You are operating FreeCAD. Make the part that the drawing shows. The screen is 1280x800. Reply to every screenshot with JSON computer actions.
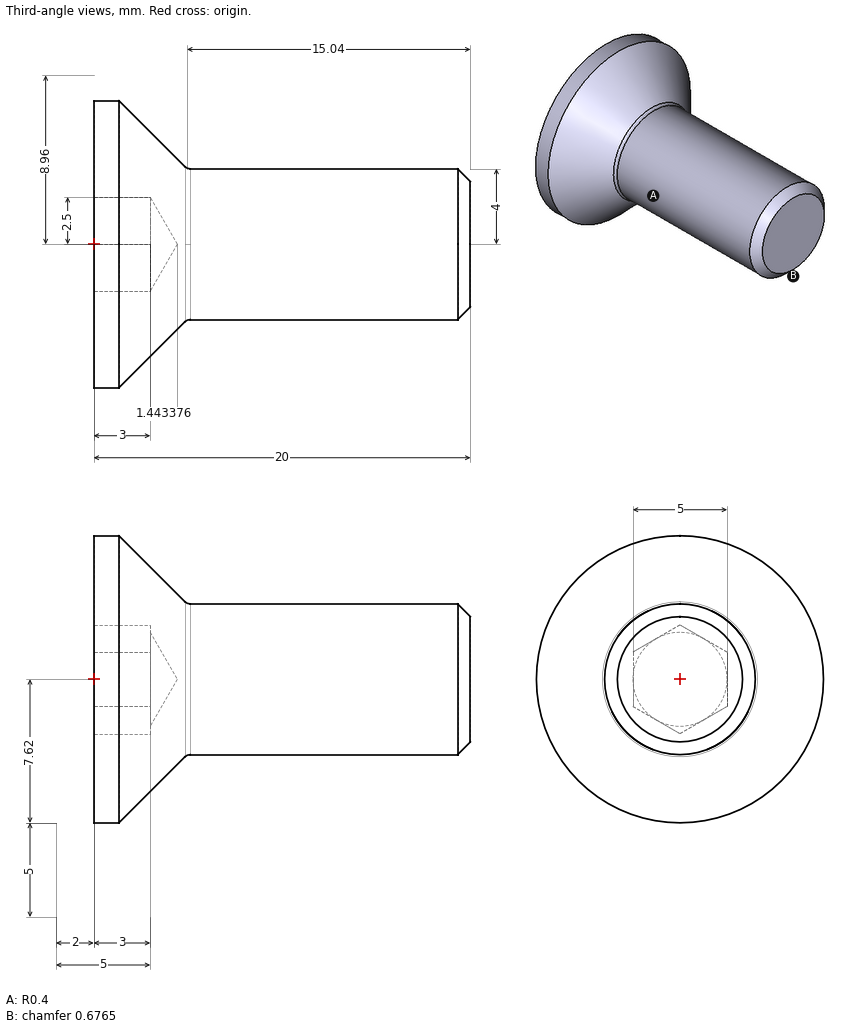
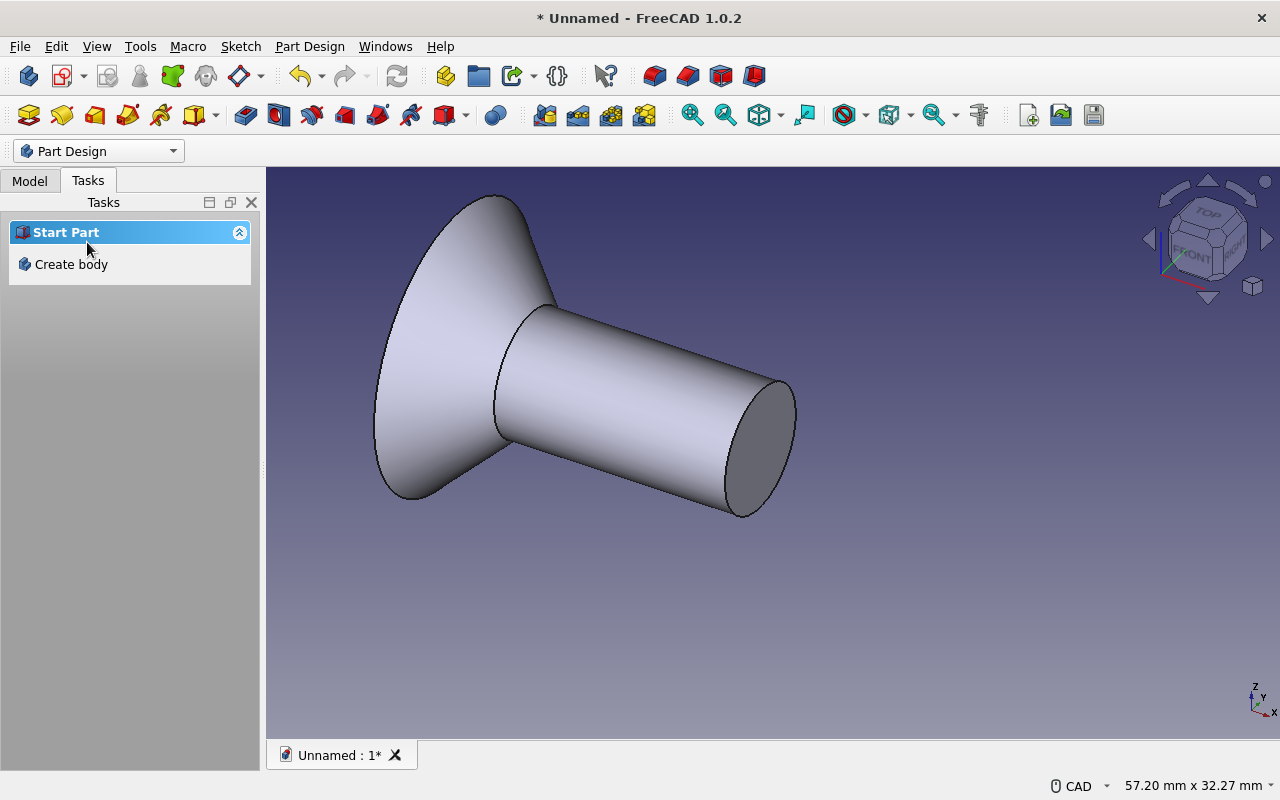
{"action": "left_click", "coordinate": [693, 116]}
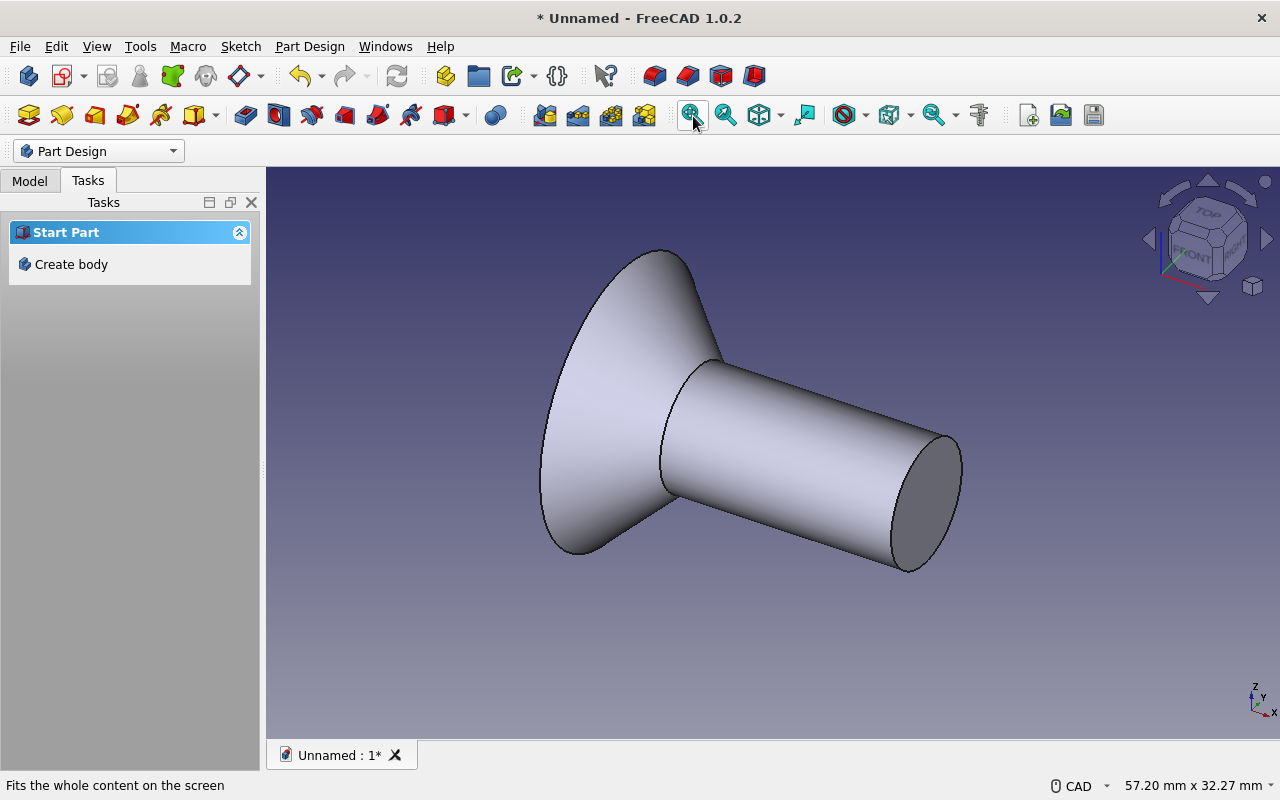
{"action": "key", "text": "0"}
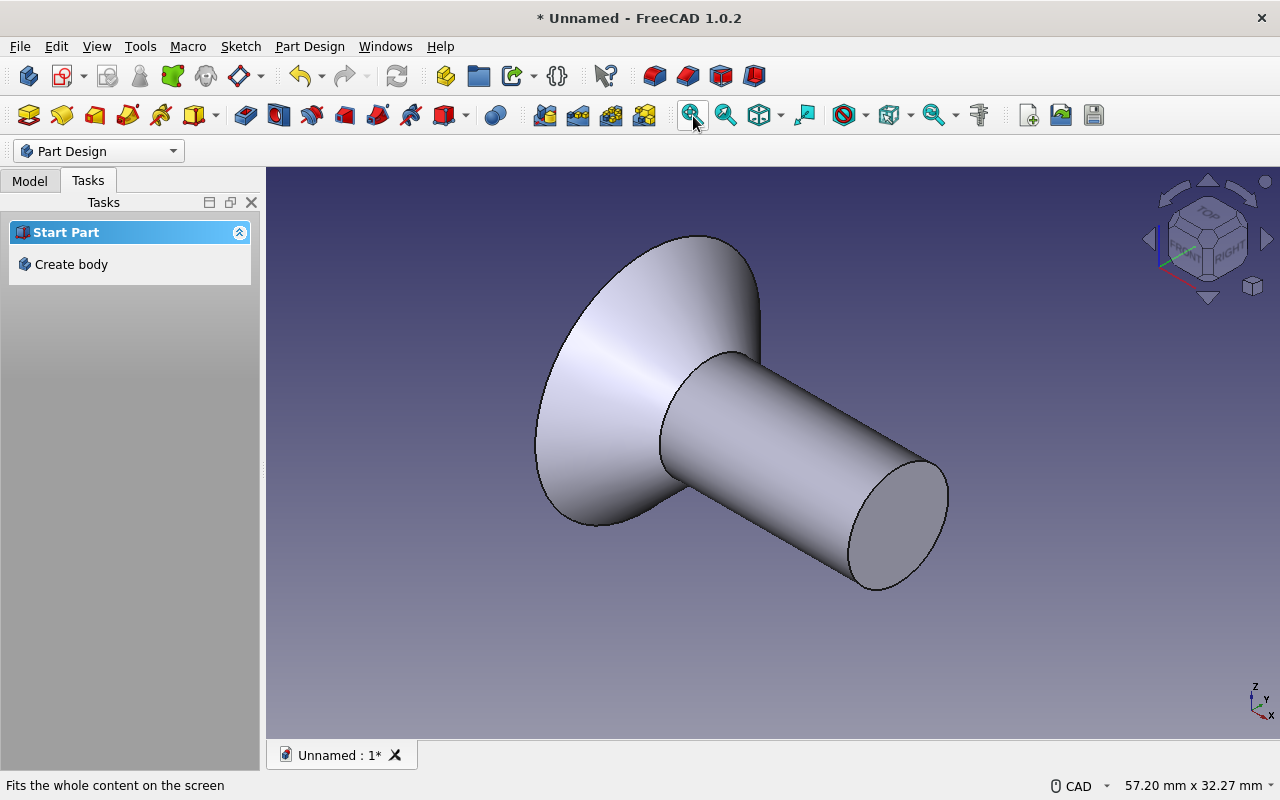
{"action": "key", "text": "2"}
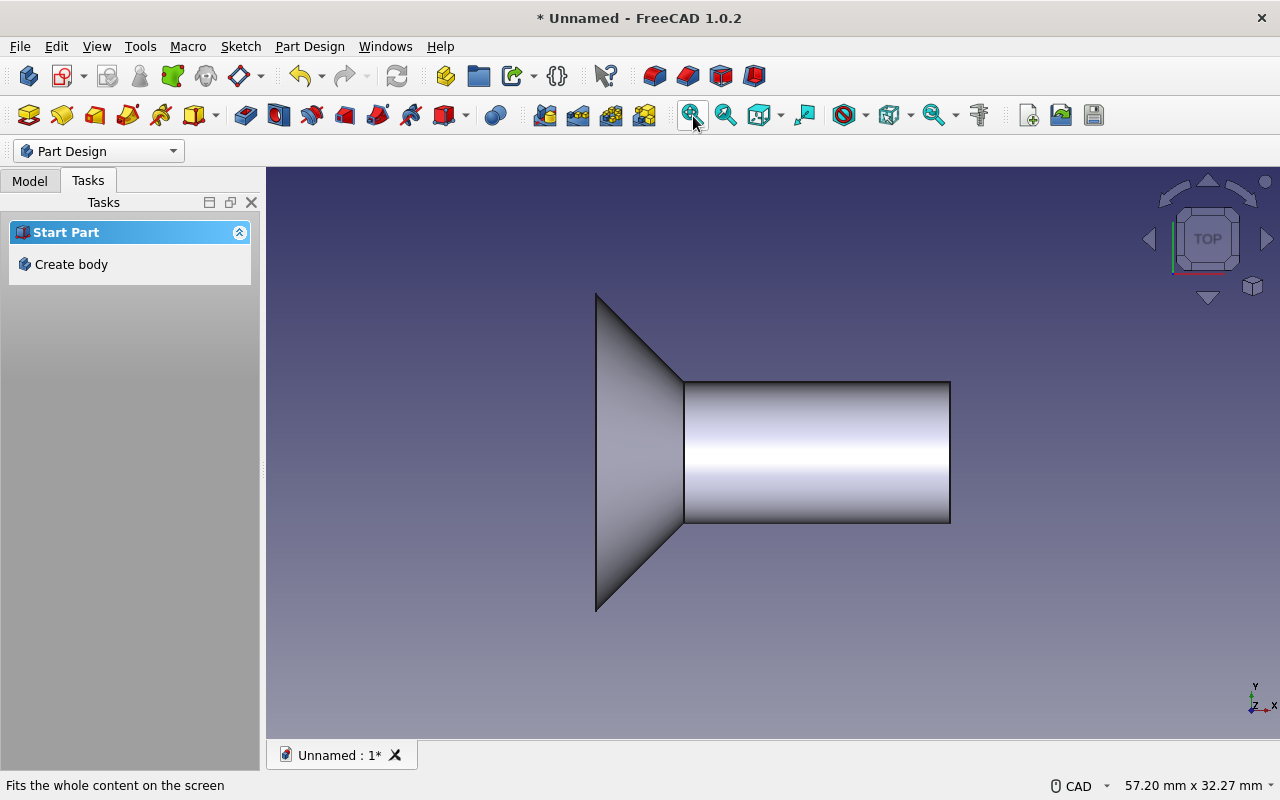
{"action": "left_click", "coordinate": [684, 510]}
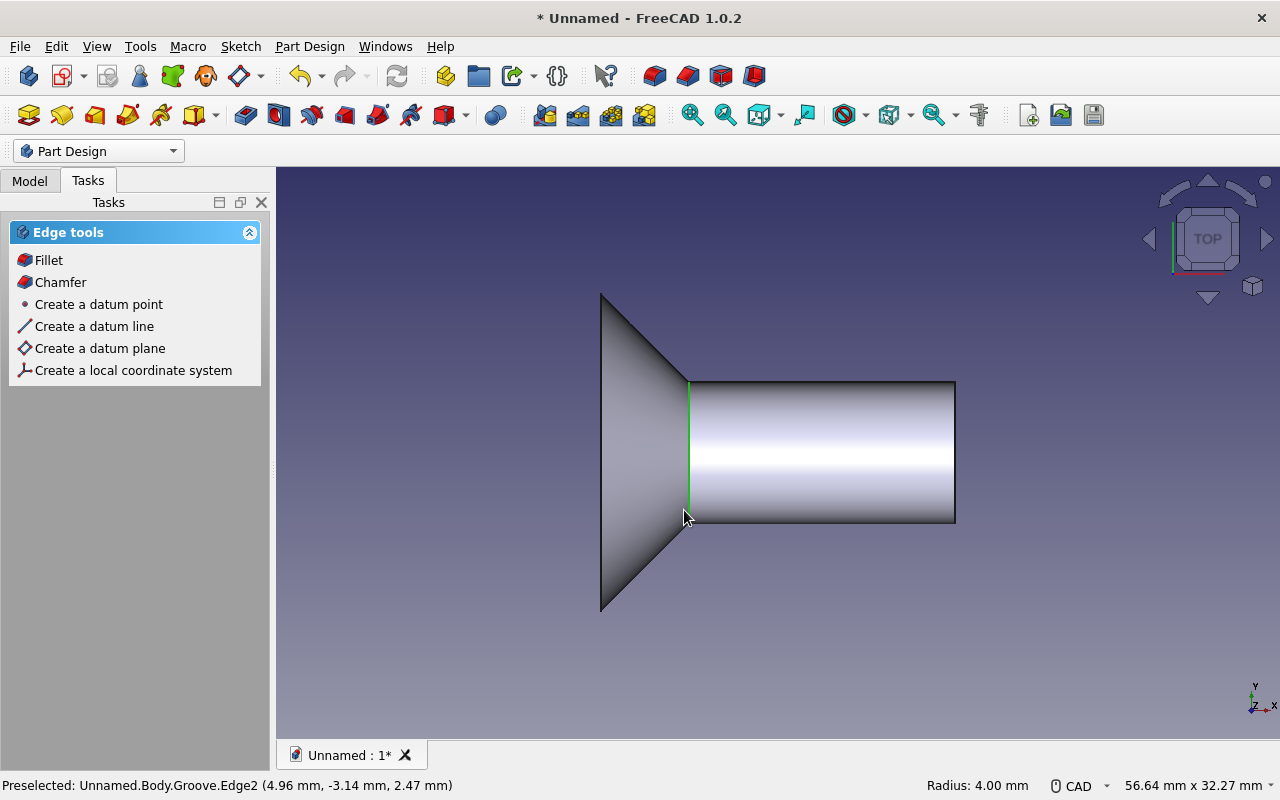
{"action": "left_click", "coordinate": [655, 76]}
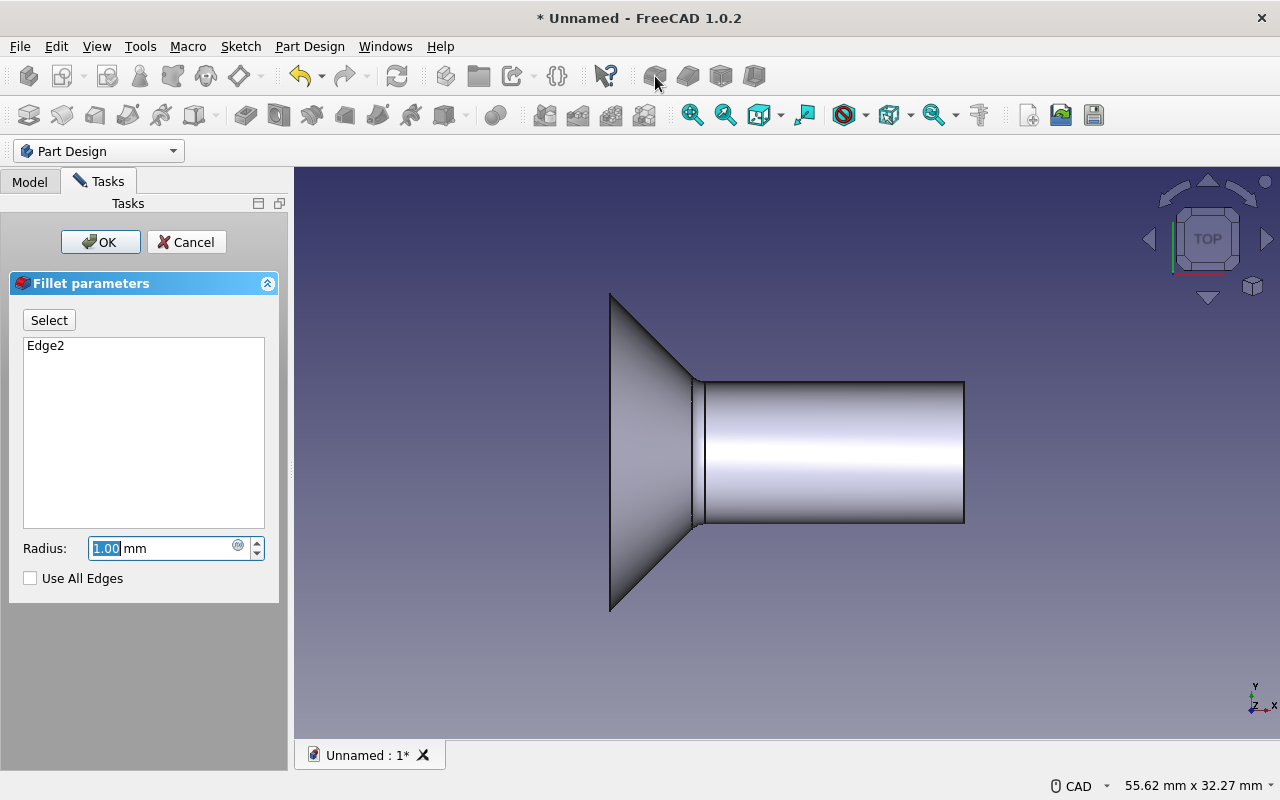
{"action": "type", "text": "0.4"}
{"action": "key", "text": "Tab"}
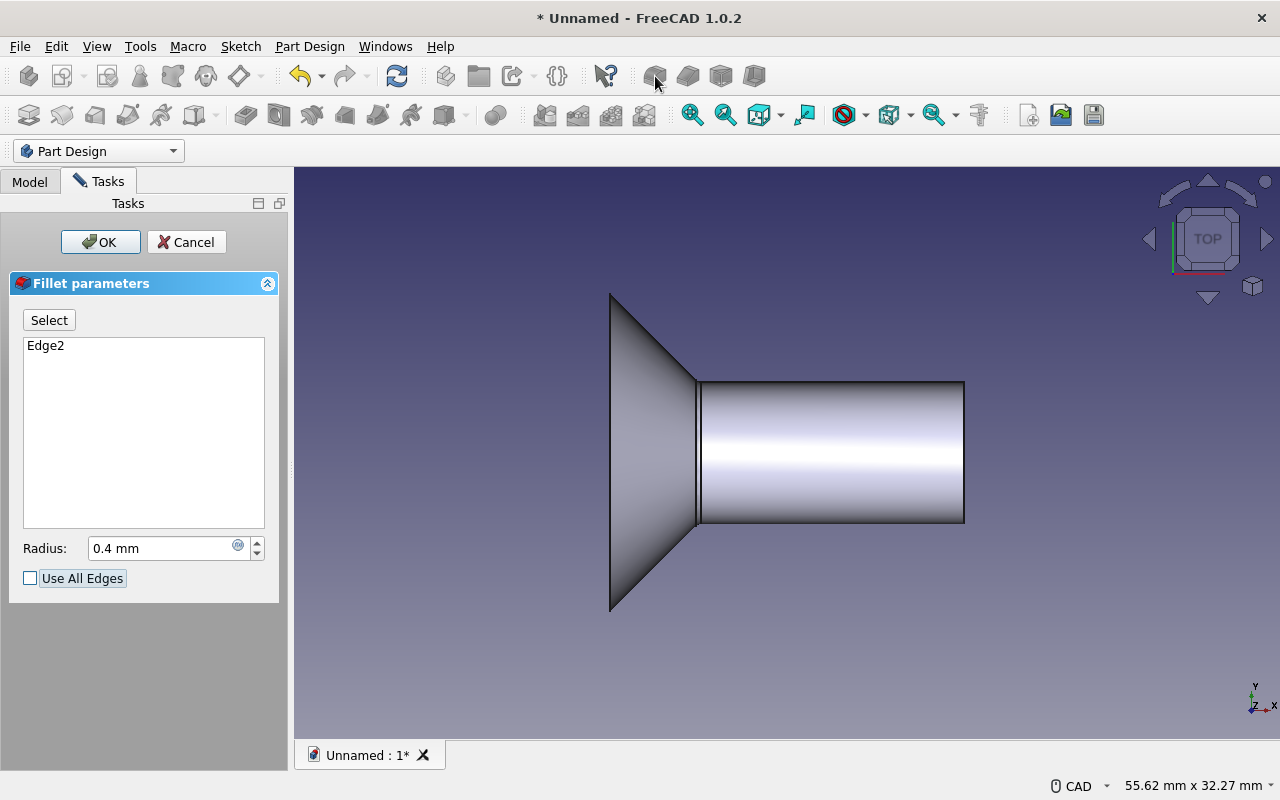
{"action": "left_click", "coordinate": [101, 242]}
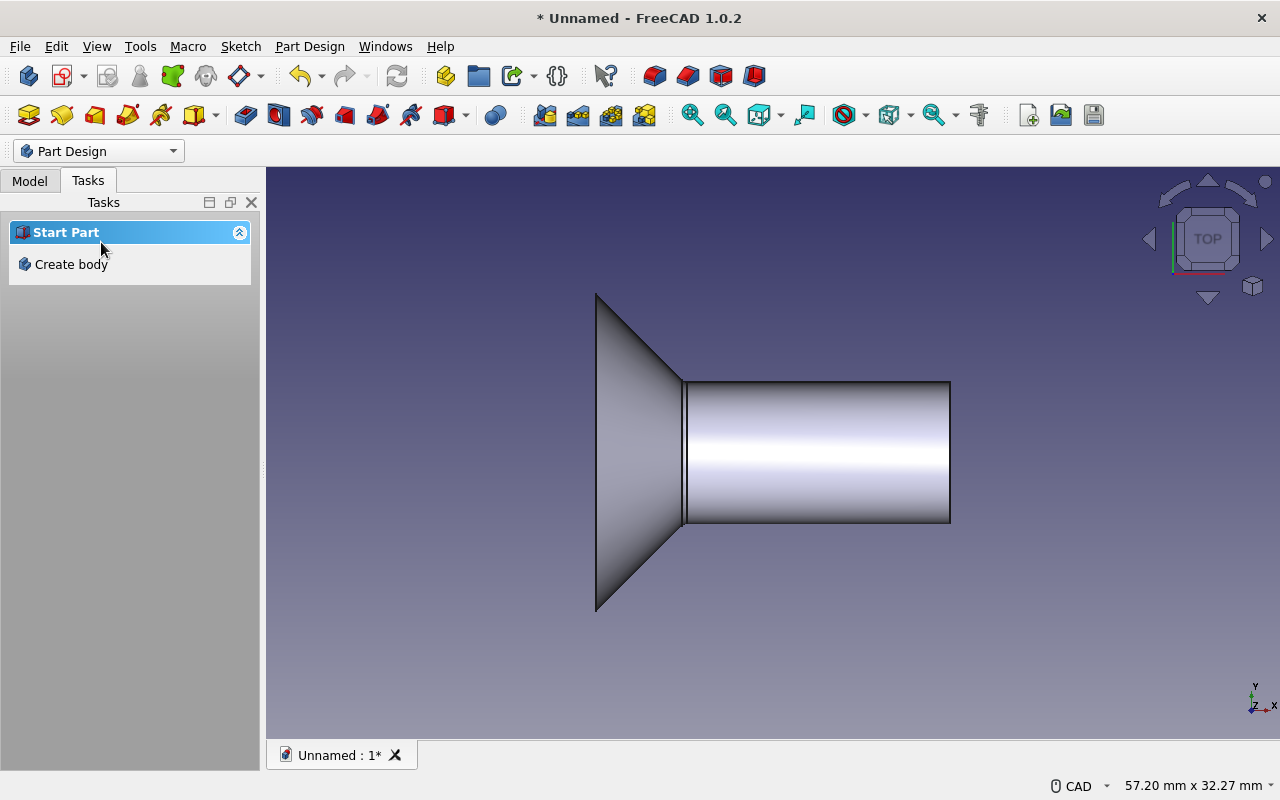
{"action": "left_click", "coordinate": [950, 510]}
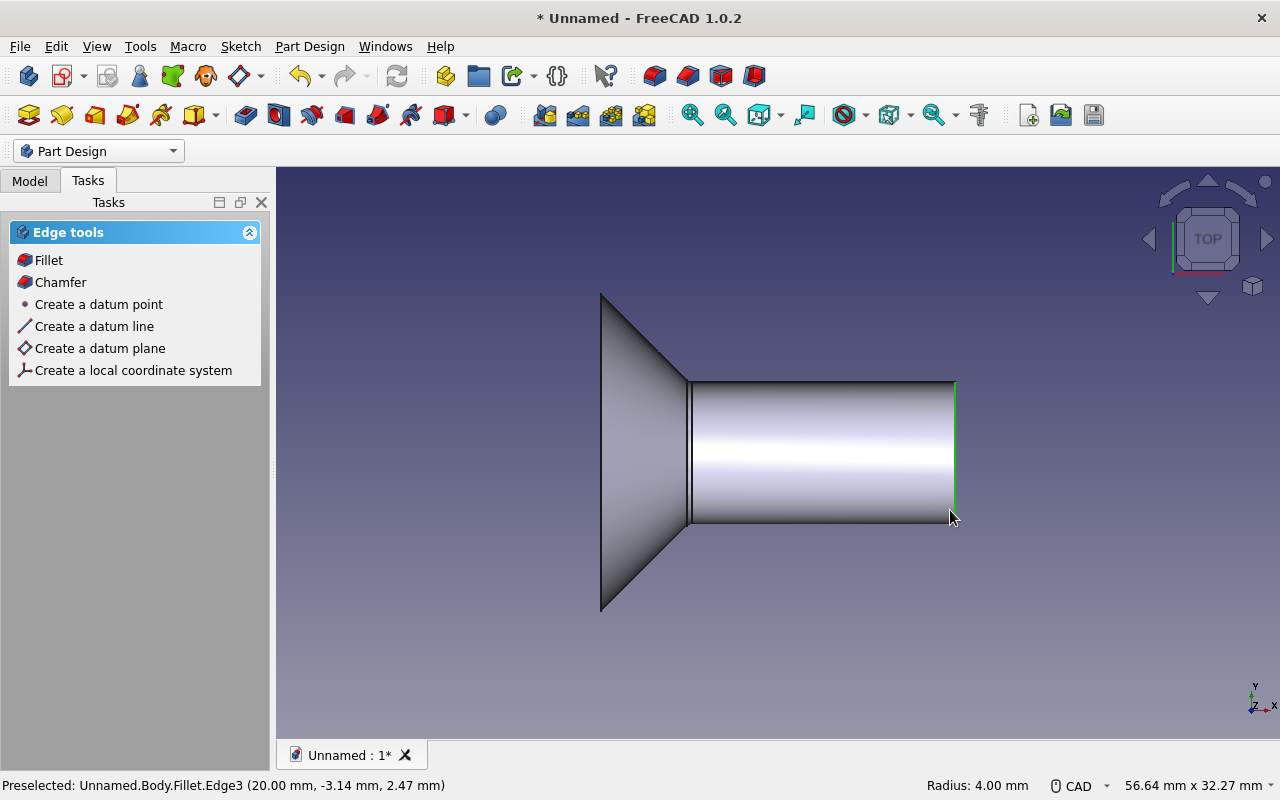
{"action": "left_click", "coordinate": [688, 76]}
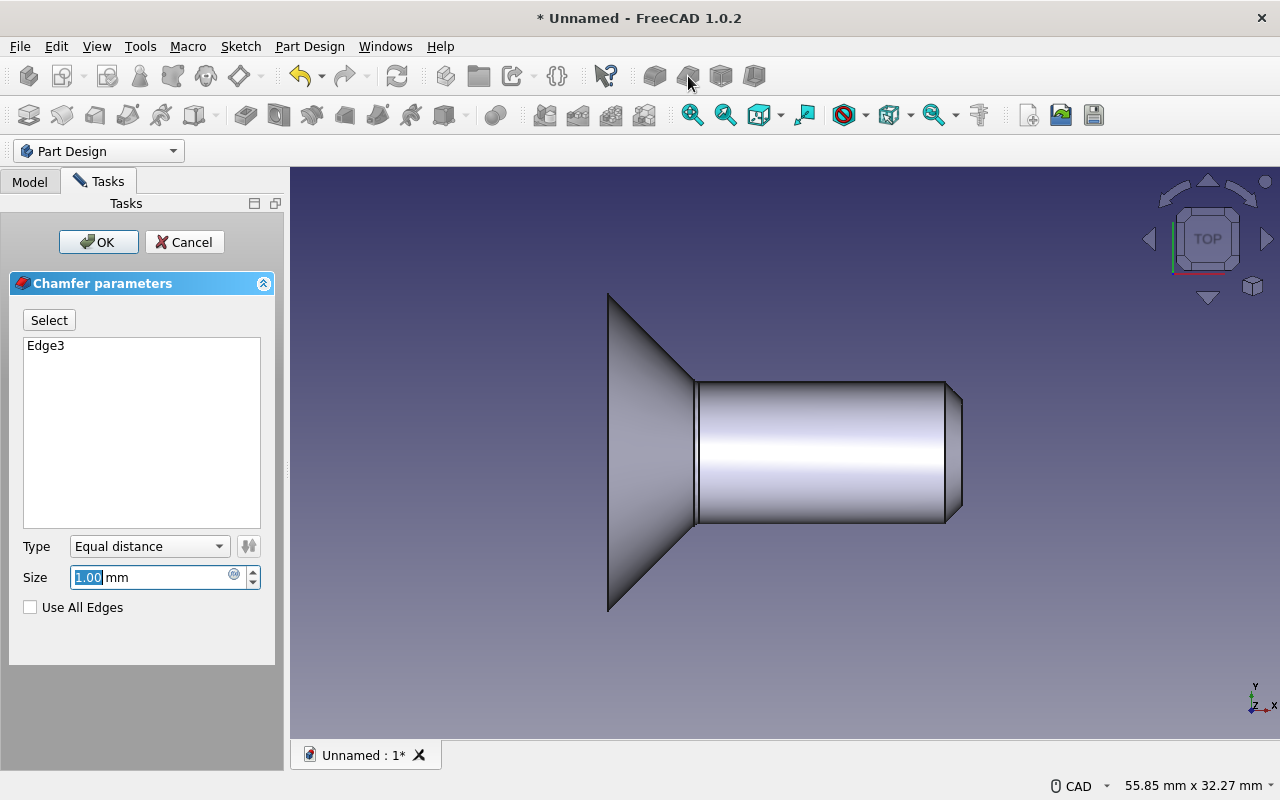
{"action": "type", "text": "0.6765"}
{"action": "key", "text": "Tab"}